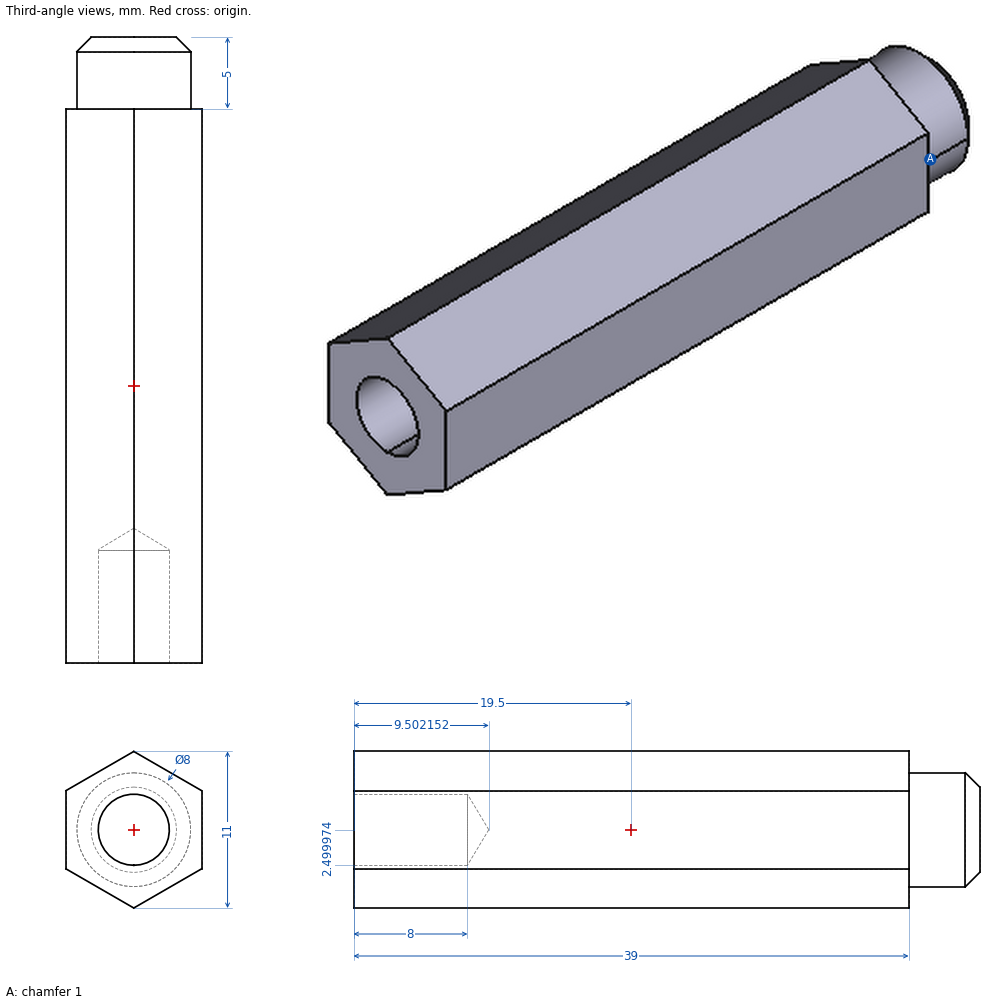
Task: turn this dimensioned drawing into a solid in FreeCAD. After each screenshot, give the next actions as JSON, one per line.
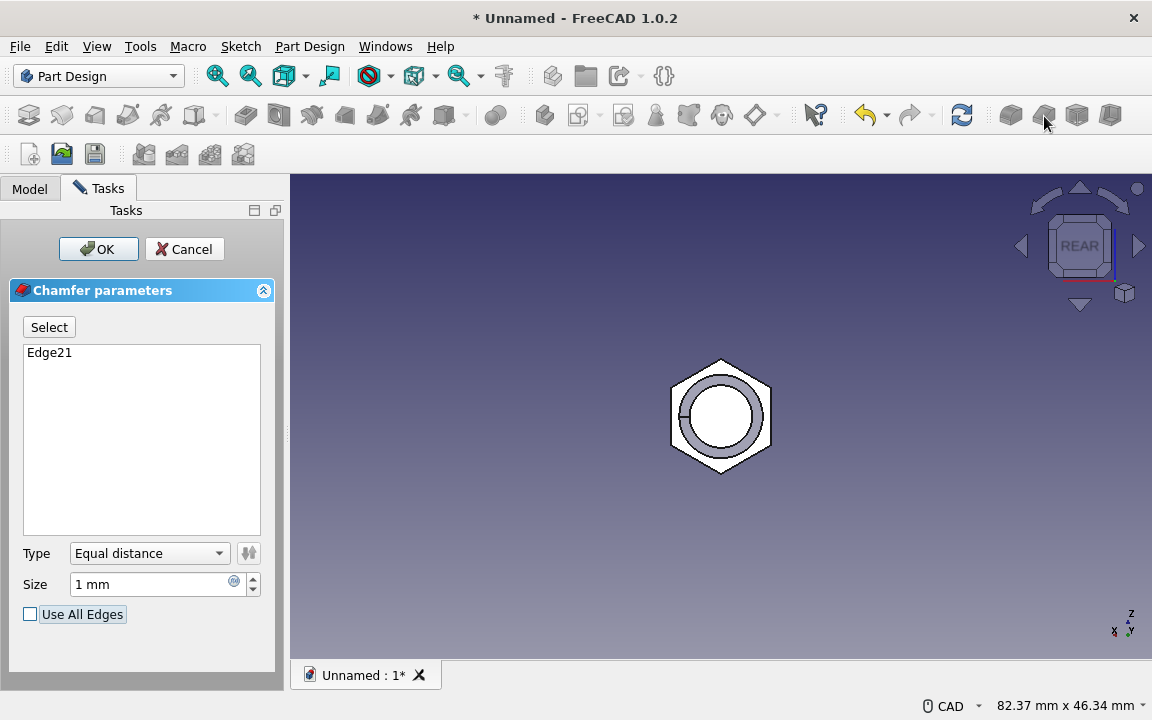
{"action": "left_click", "coordinate": [99, 249]}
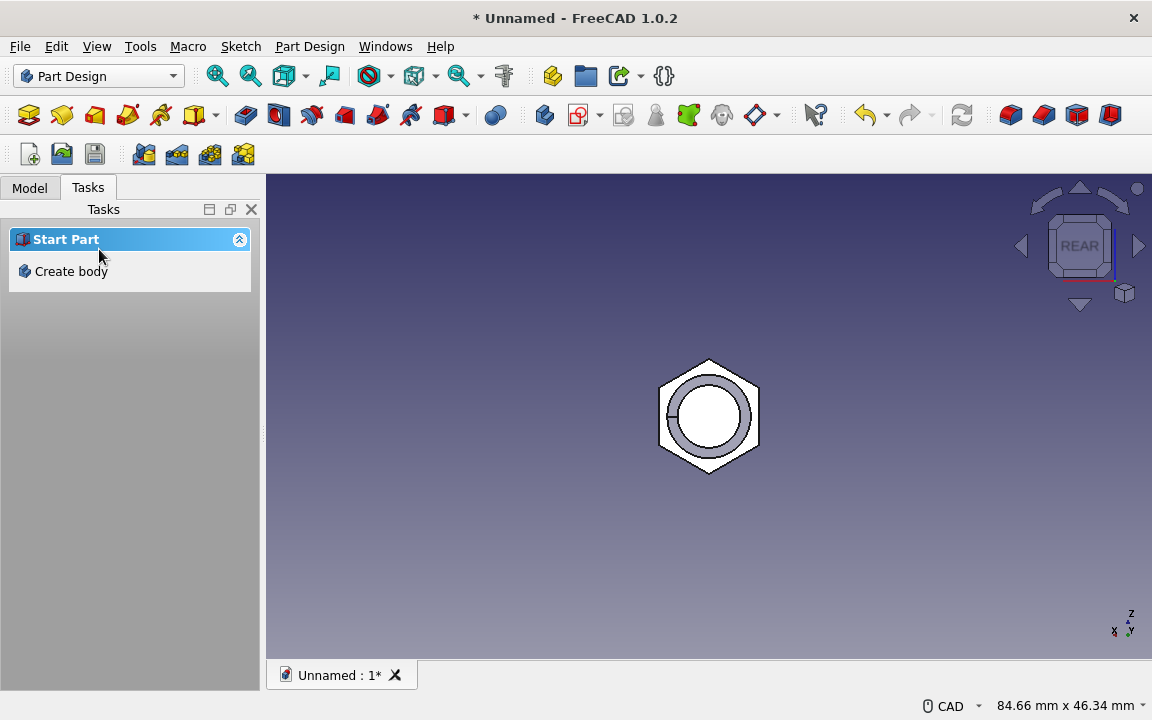
{"action": "key", "text": "v f"}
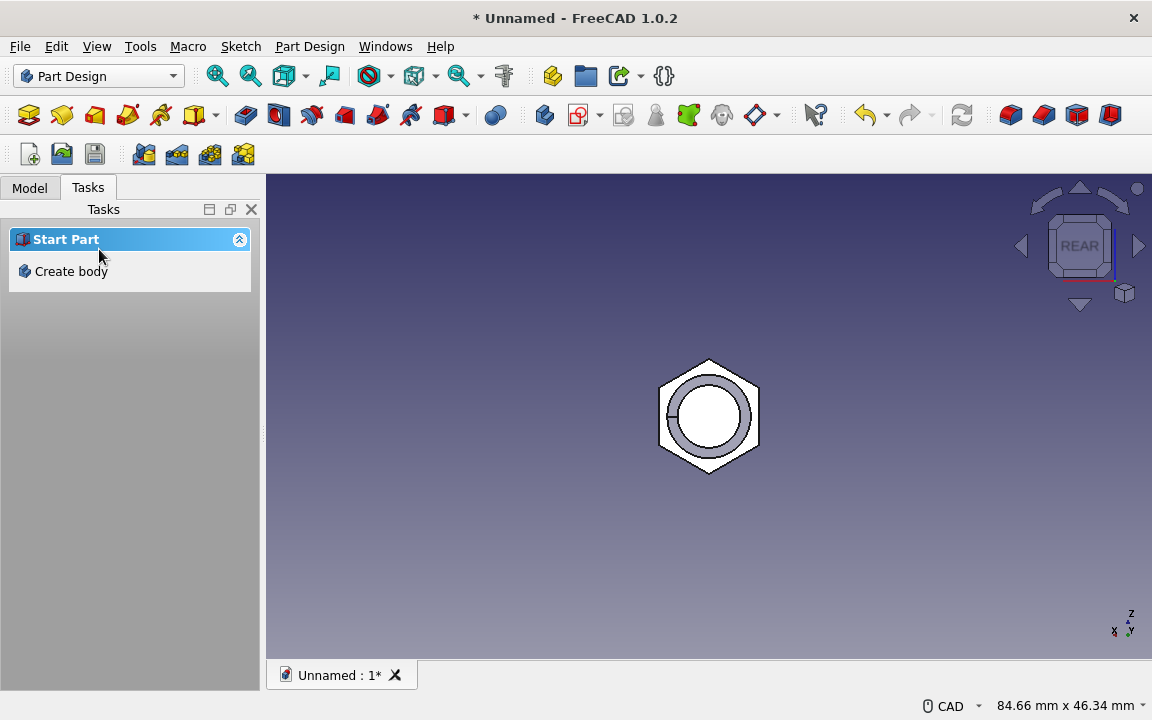
{"action": "left_click", "coordinate": [30, 188]}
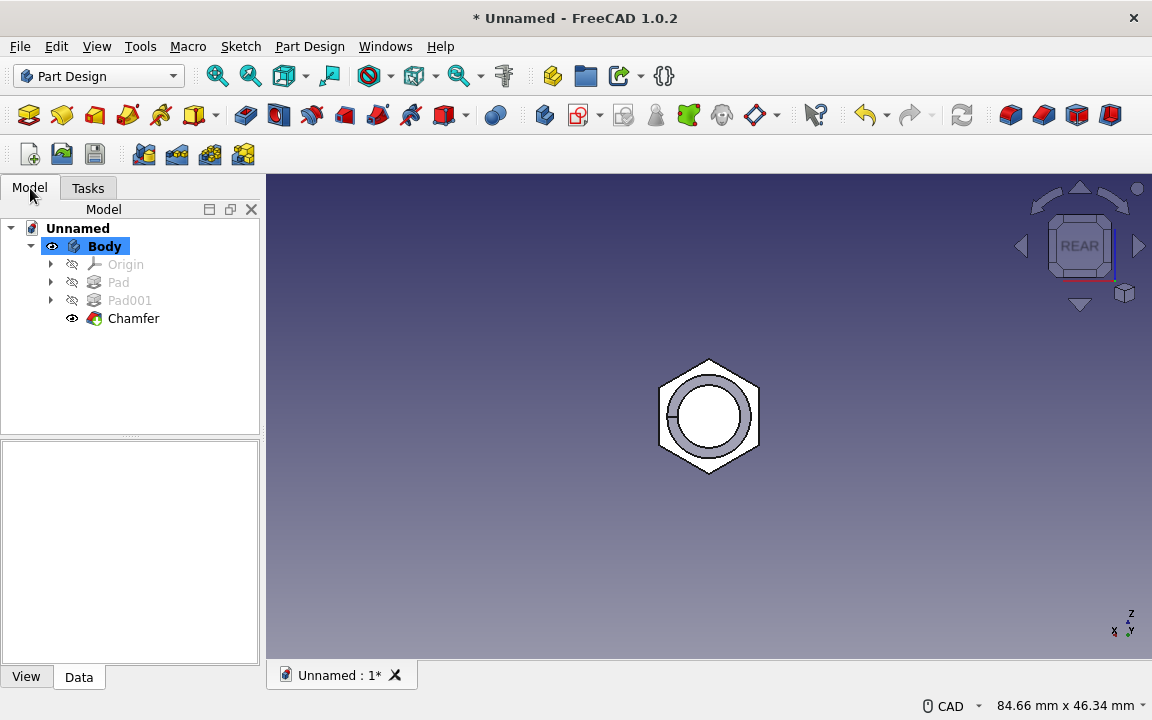
{"action": "left_click", "coordinate": [51, 264]}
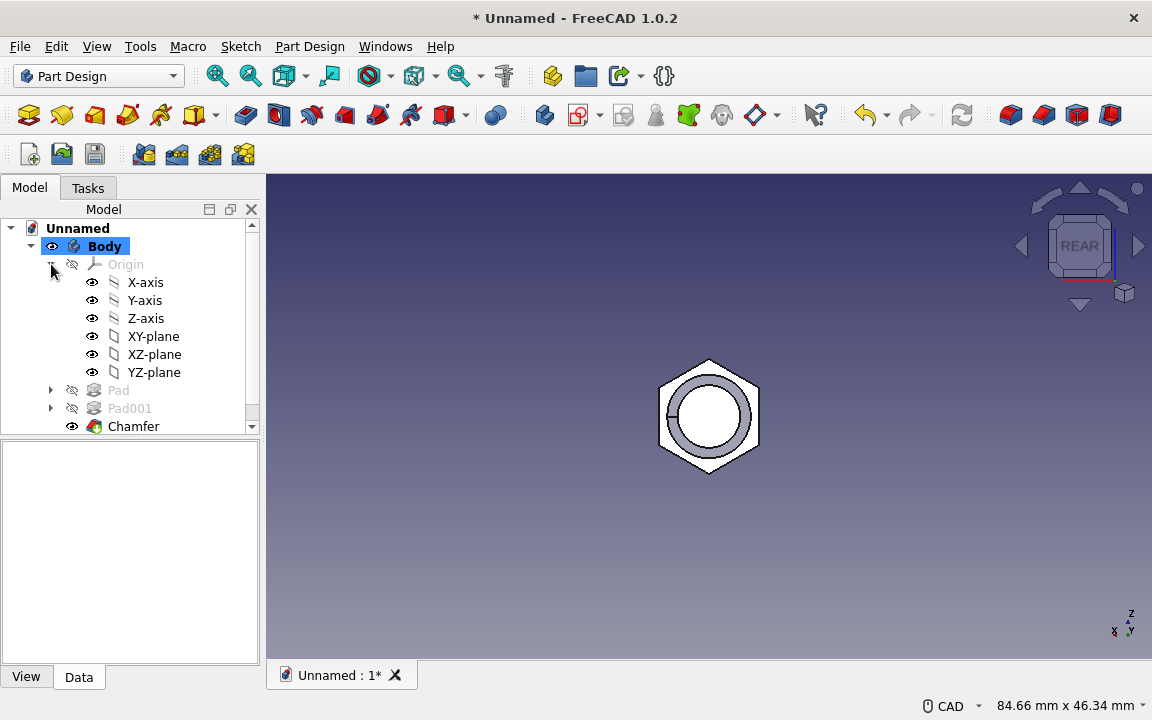
{"action": "left_click", "coordinate": [137, 372]}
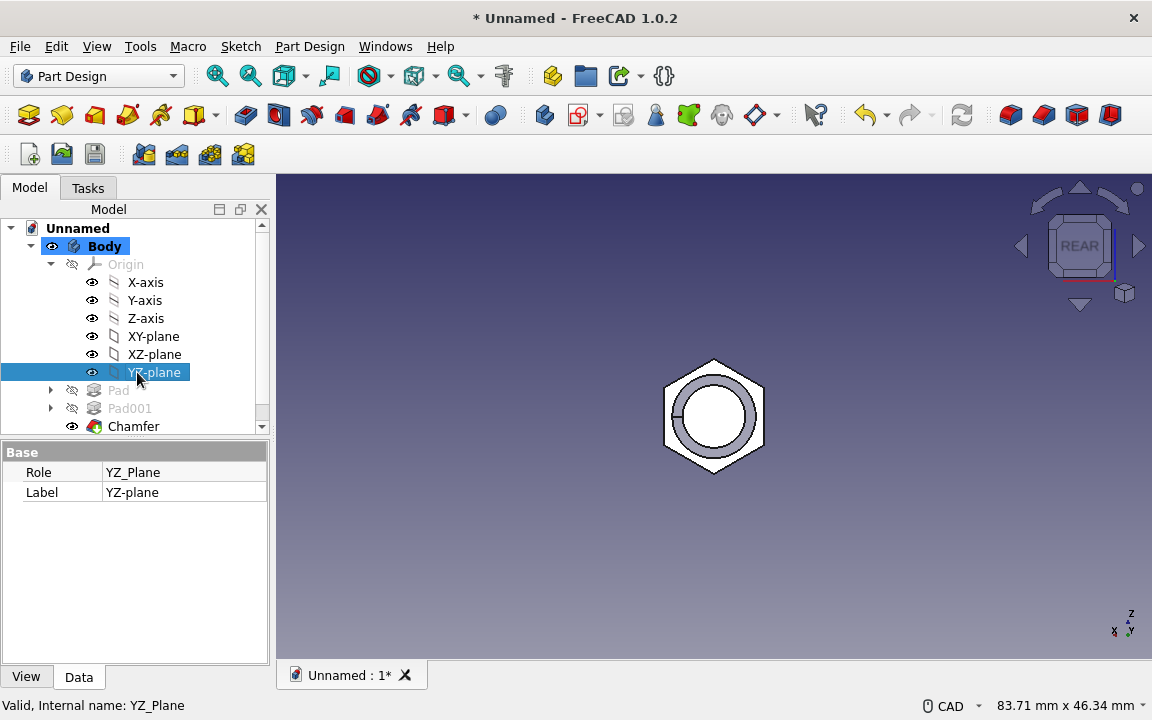
{"action": "left_click", "coordinate": [754, 116]}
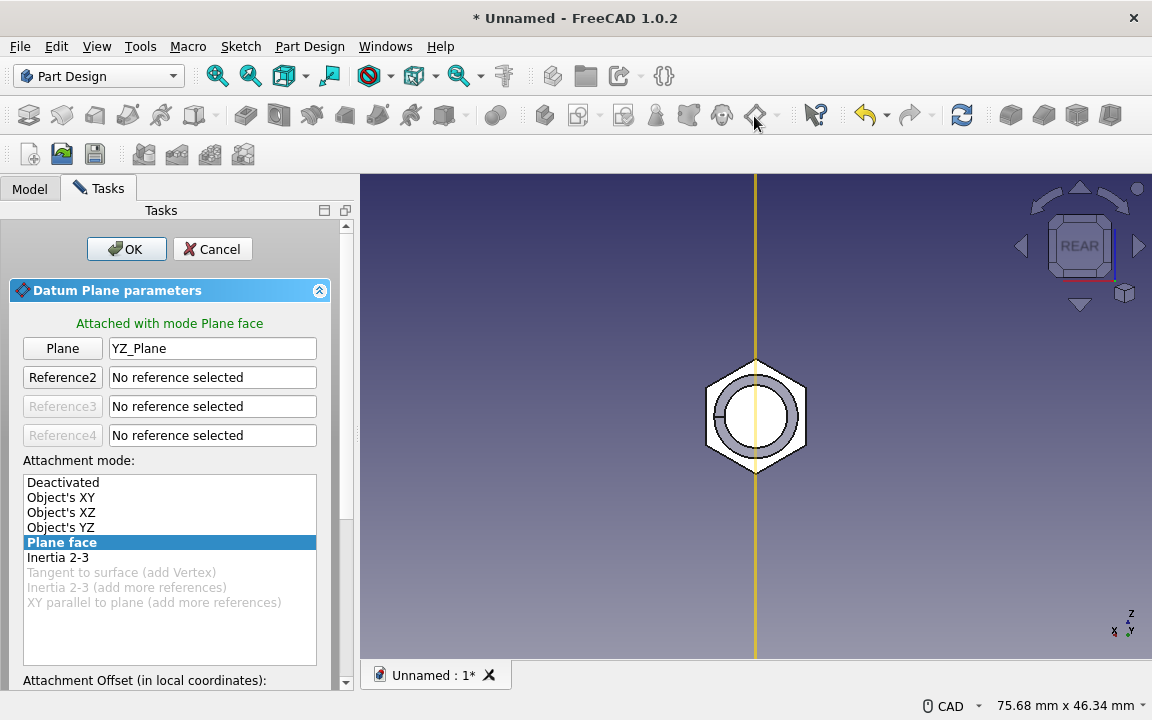
{"action": "scroll", "coordinate": [346, 455], "scroll_direction": "down", "scroll_amount": 3}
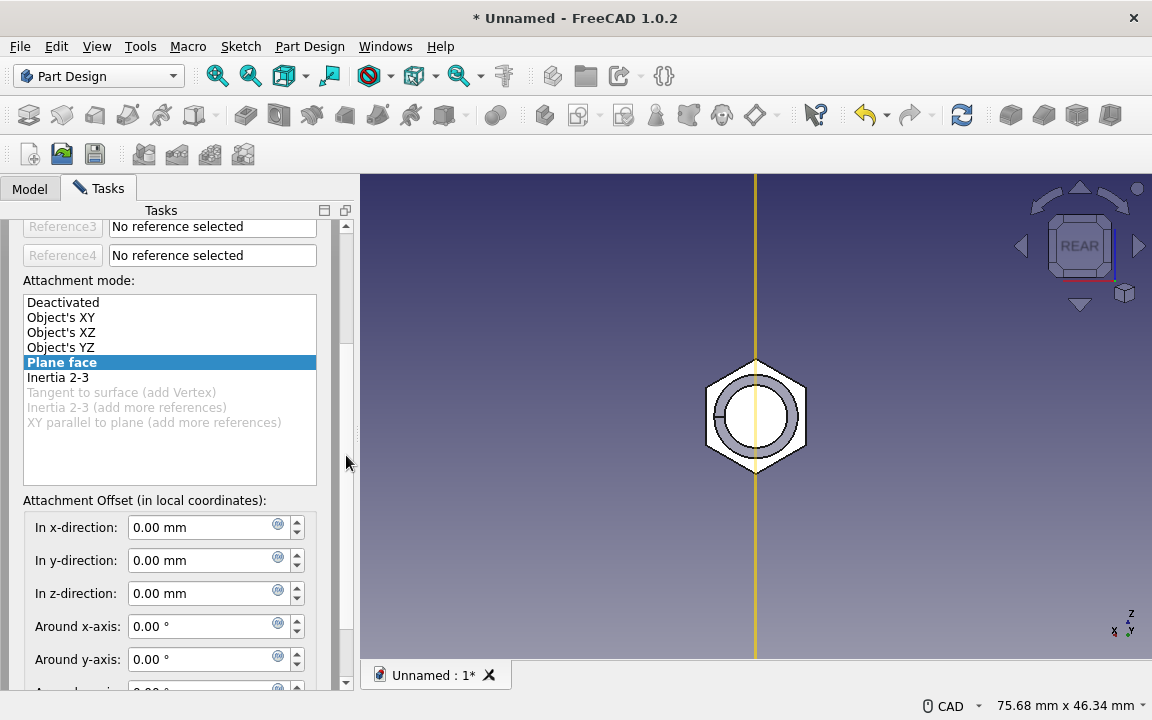
{"action": "triple_click", "coordinate": [210, 594]}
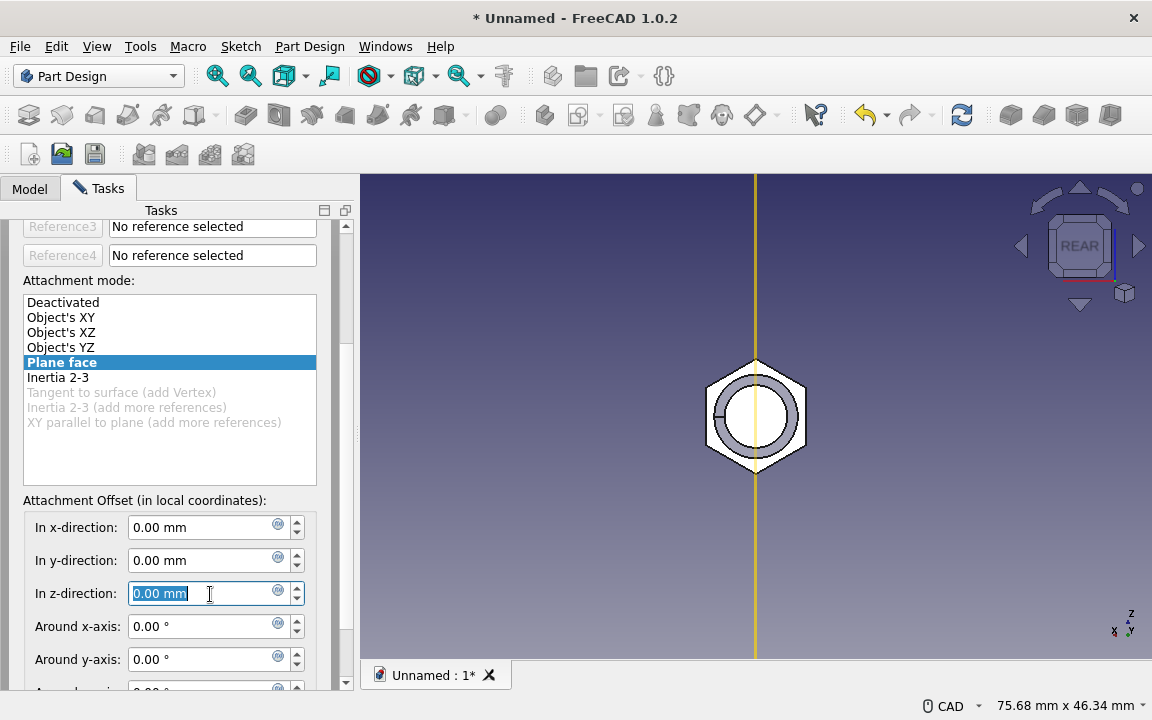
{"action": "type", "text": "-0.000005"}
{"action": "key", "text": "Tab"}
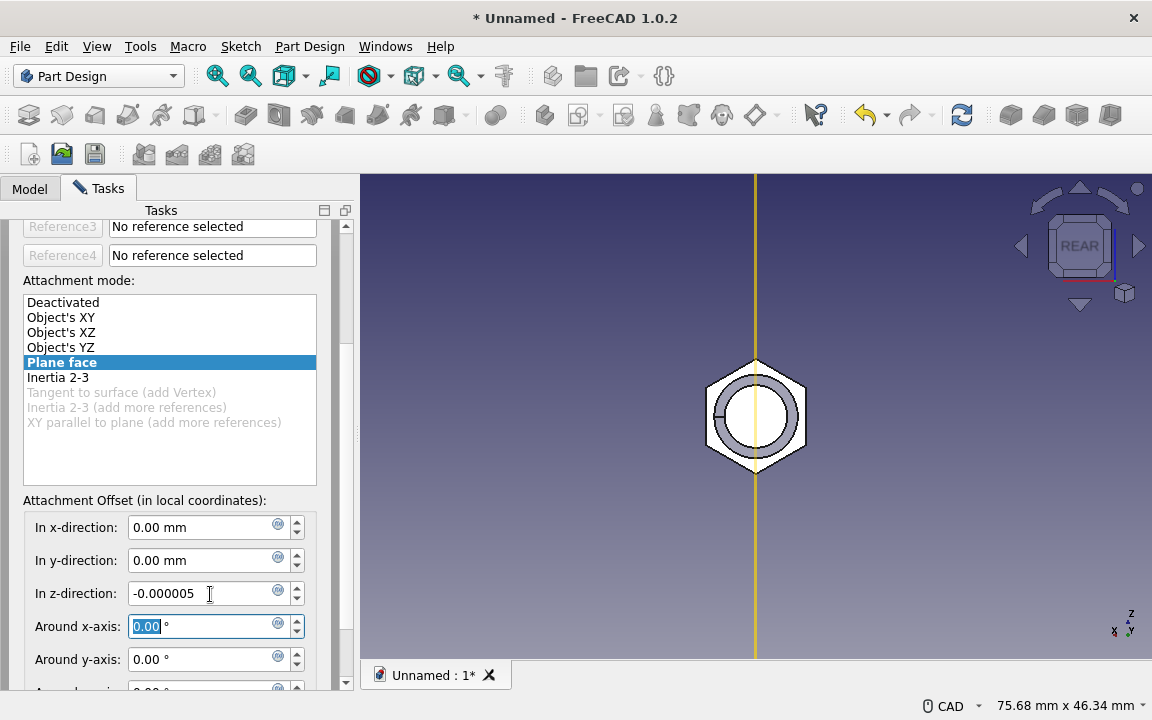
{"action": "scroll", "coordinate": [346, 455], "scroll_direction": "up", "scroll_amount": 4}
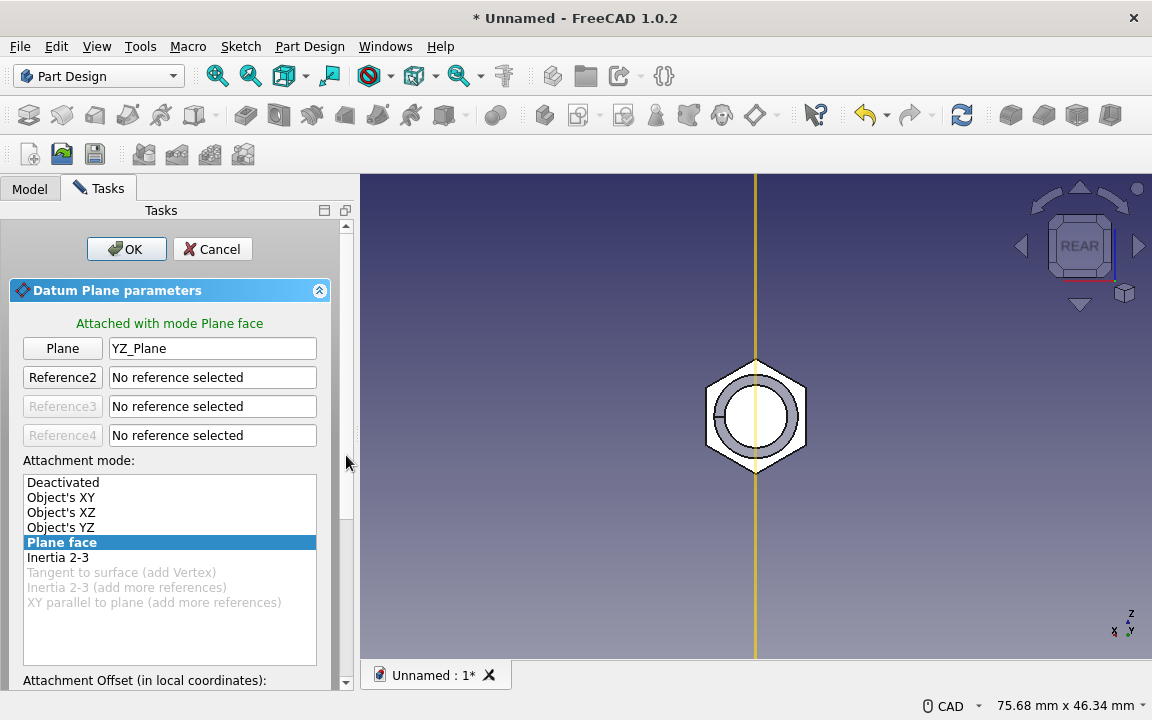
{"action": "left_click", "coordinate": [127, 249]}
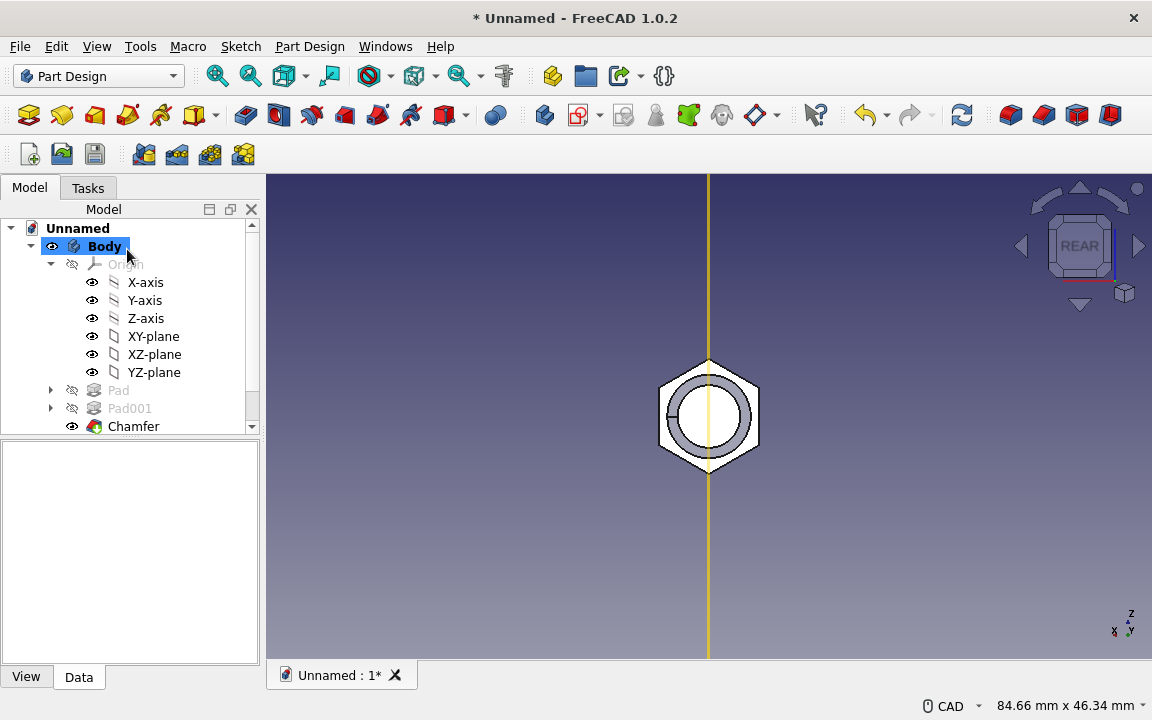
{"action": "scroll", "coordinate": [101, 332], "scroll_direction": "down", "scroll_amount": 3}